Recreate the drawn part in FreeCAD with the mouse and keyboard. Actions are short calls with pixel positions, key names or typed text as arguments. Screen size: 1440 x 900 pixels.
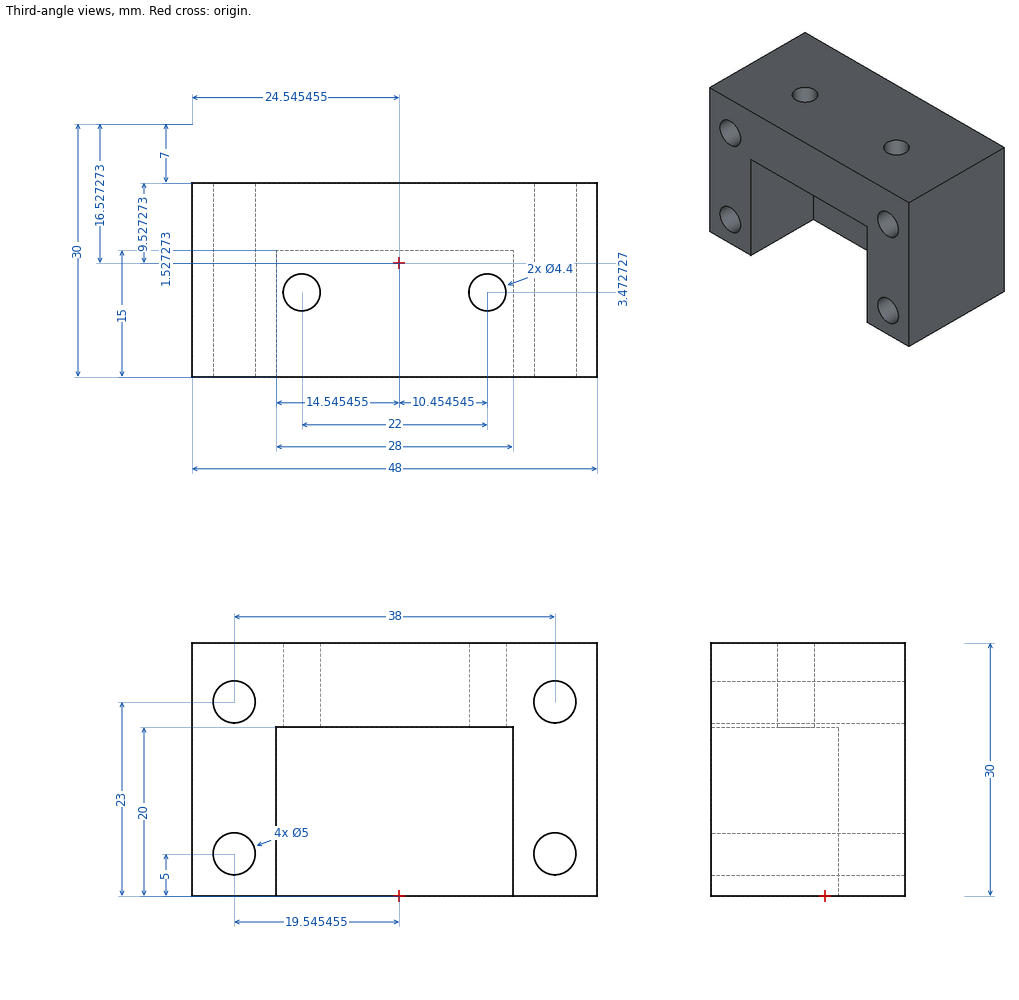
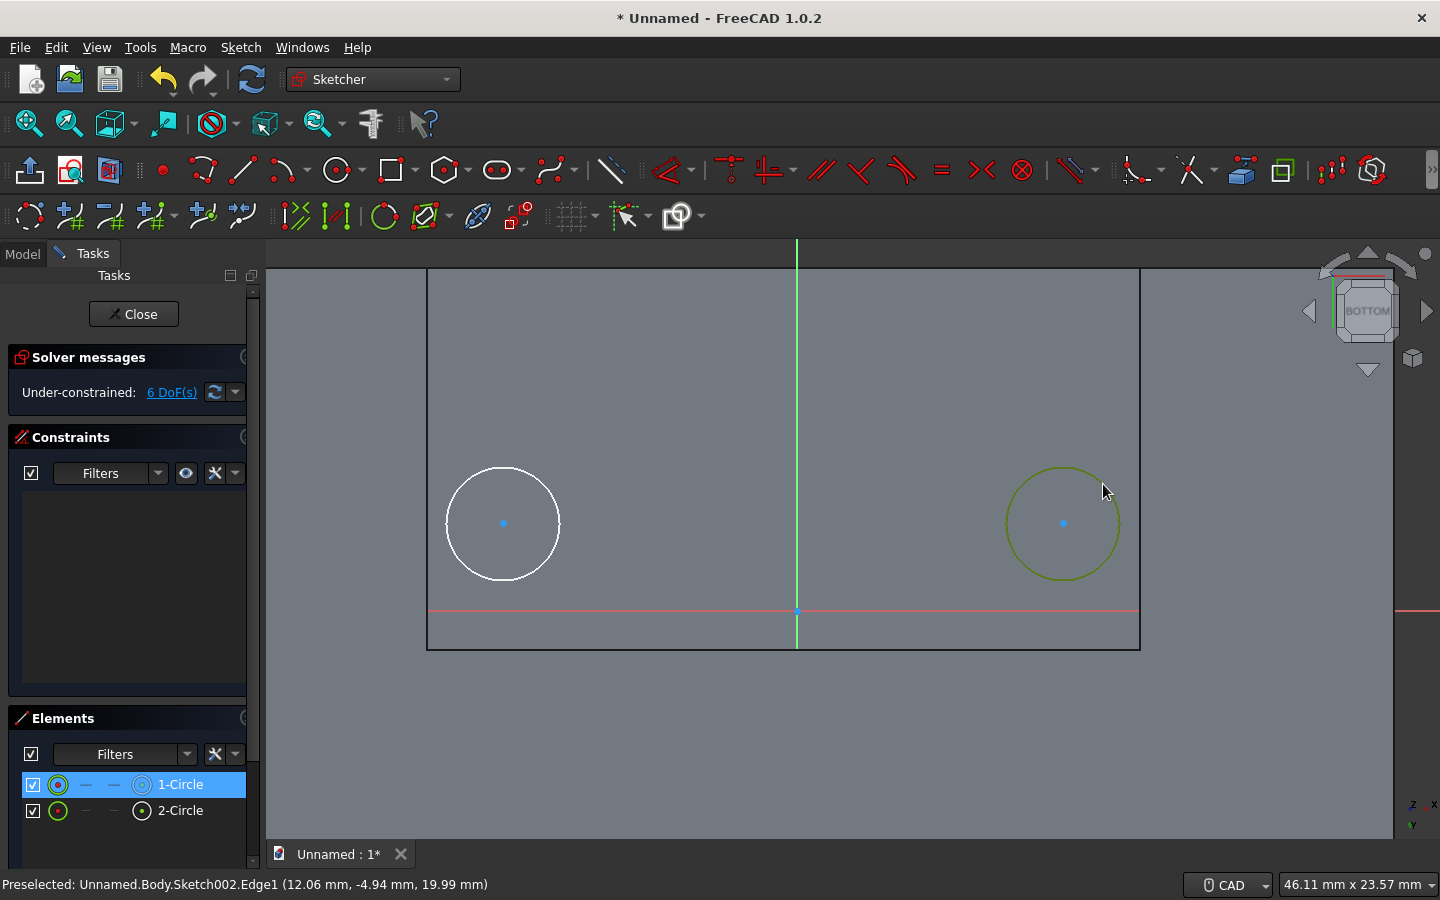
click(543, 484)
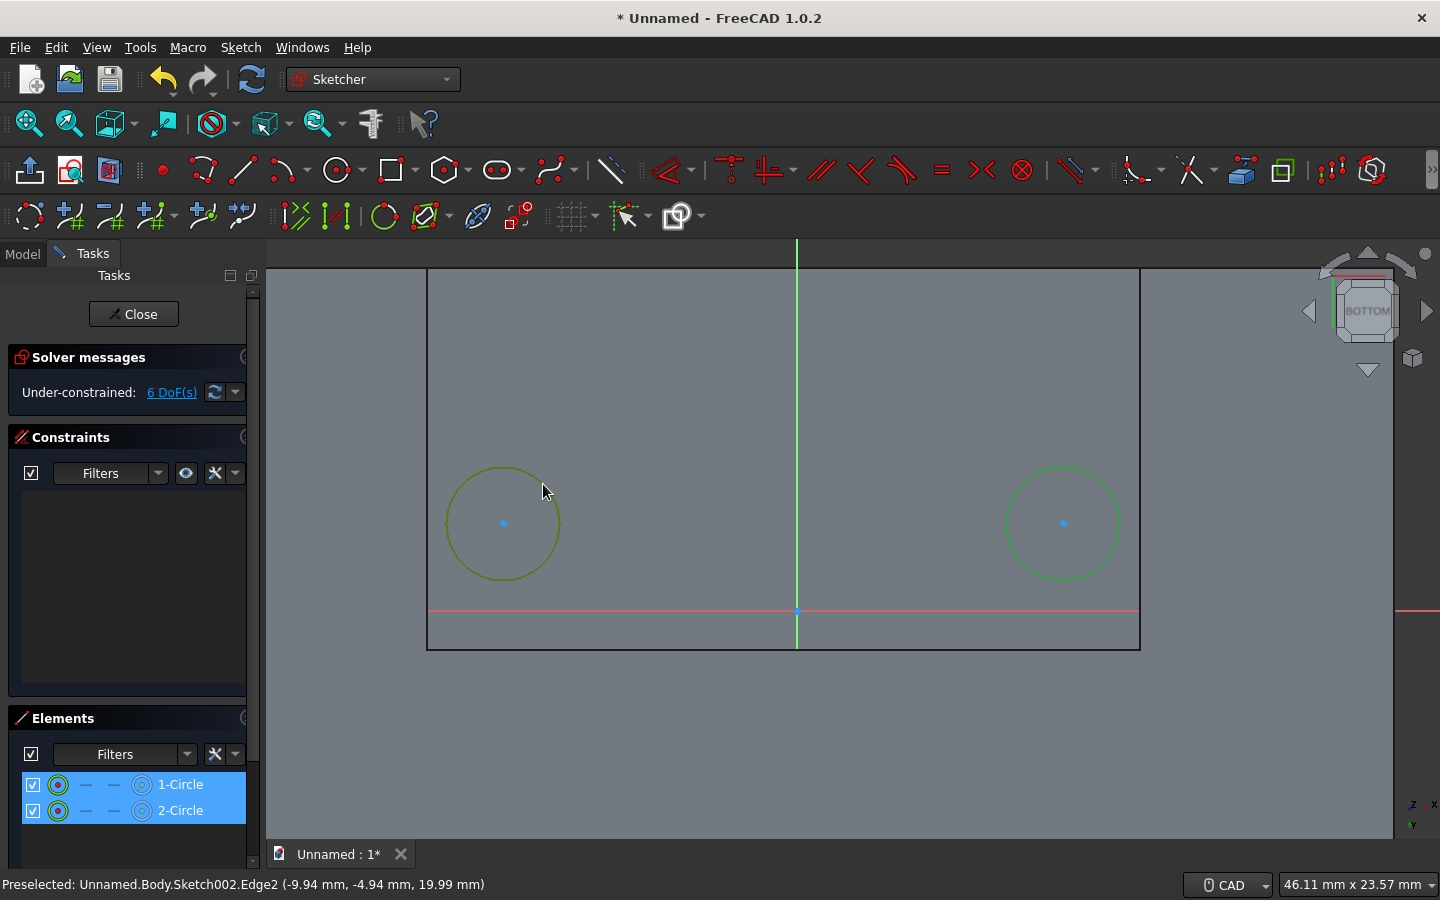
click(942, 170)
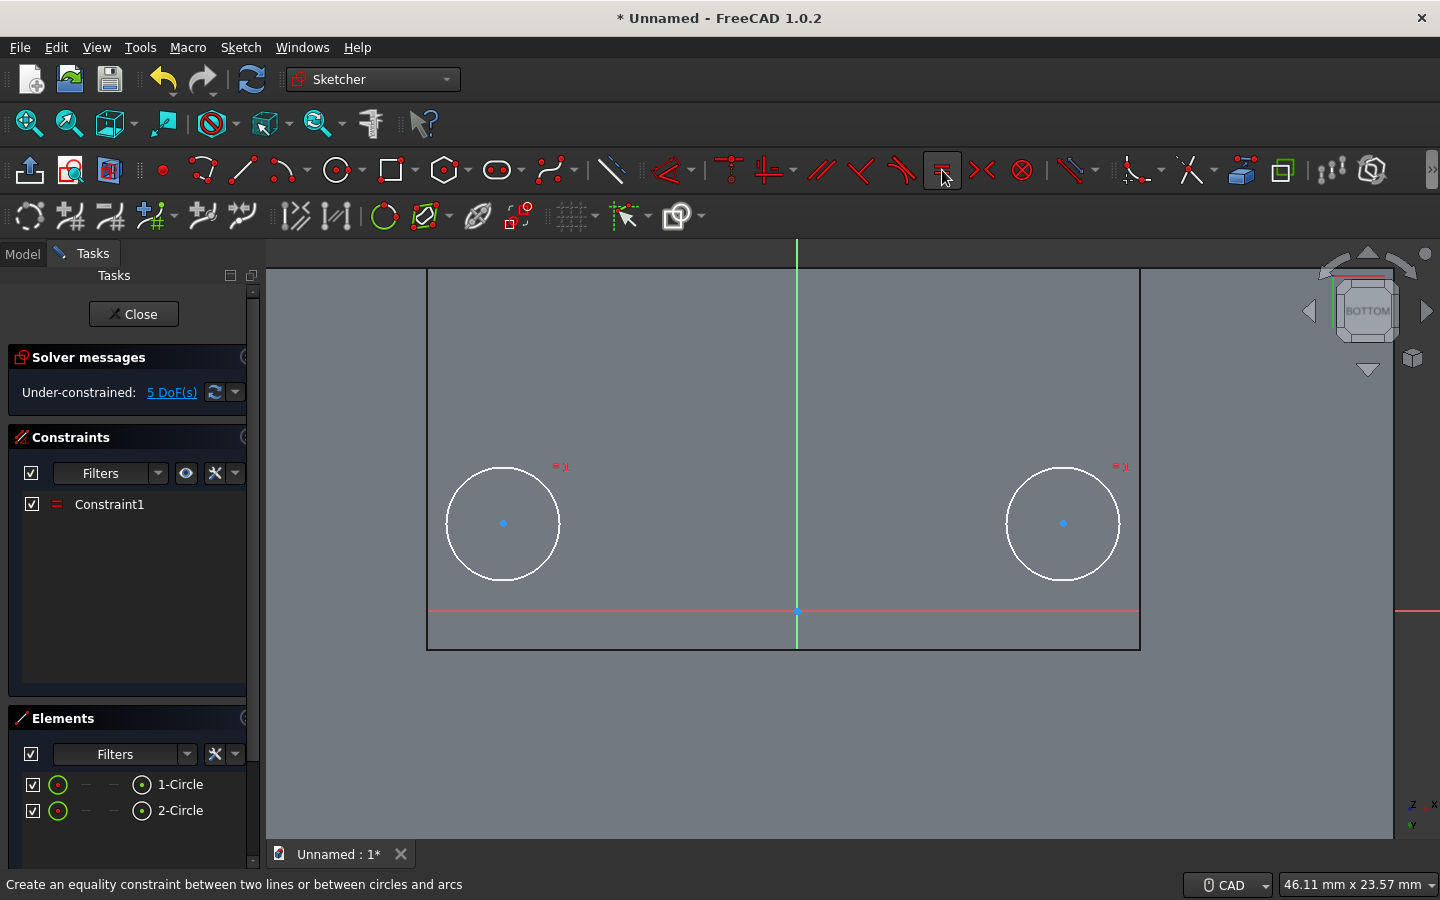
click(666, 170)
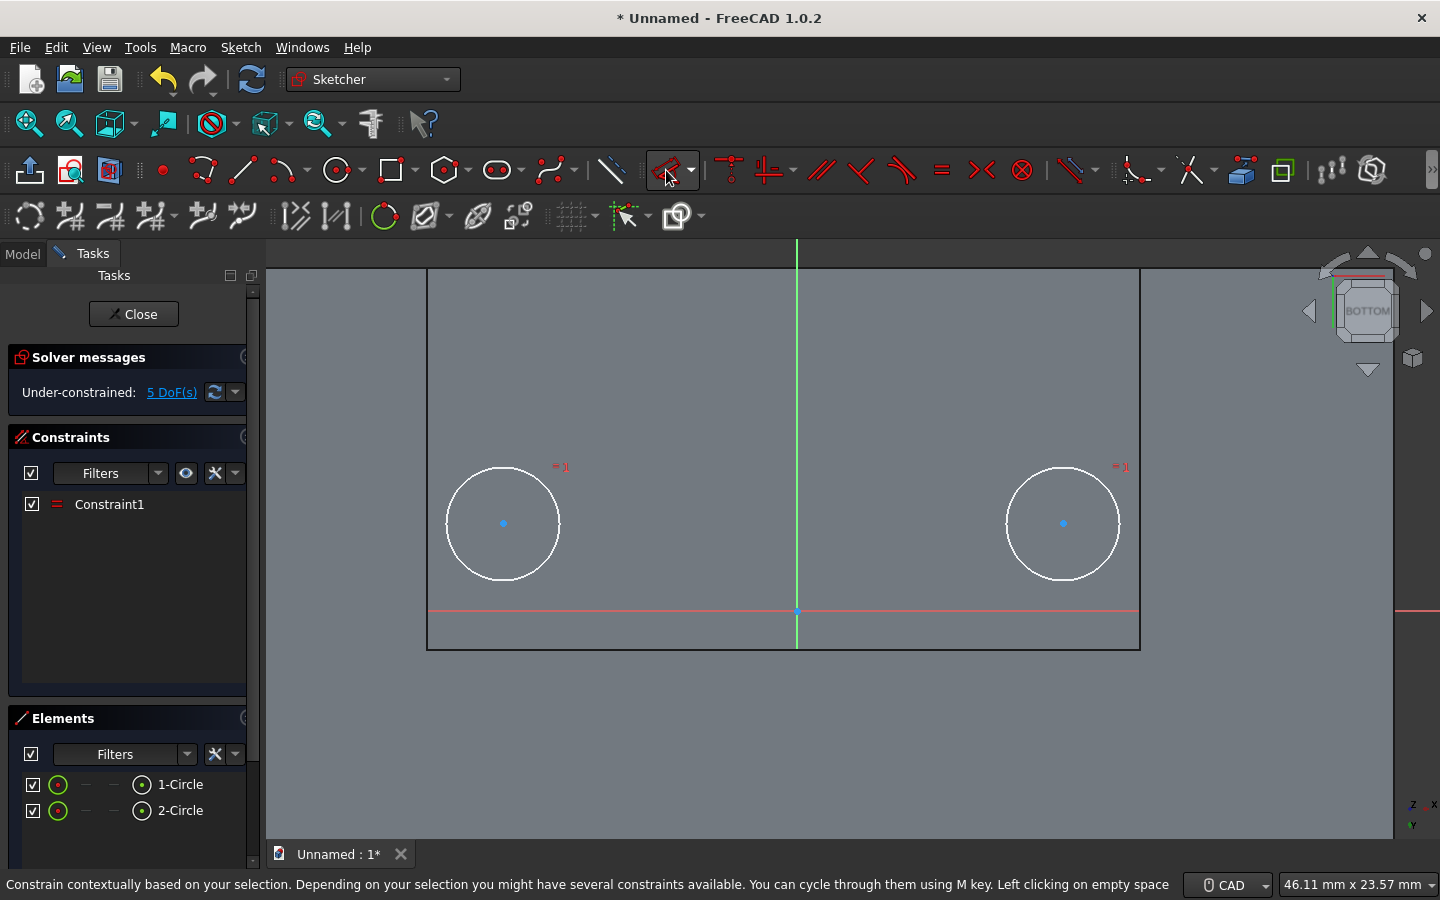
click(1103, 484)
click(1126, 461)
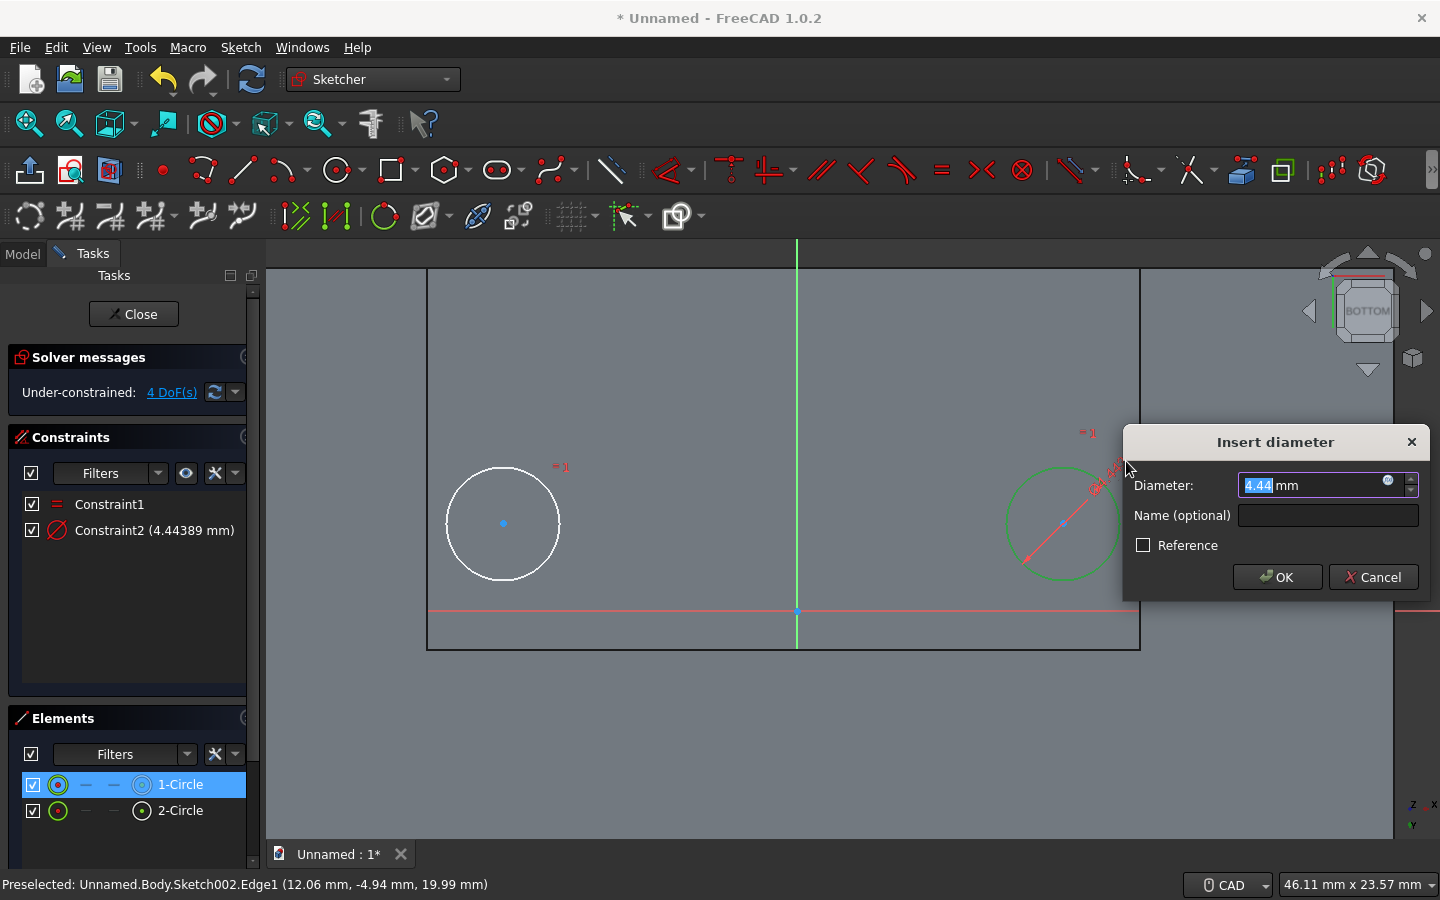
text(4.4)
key(Return)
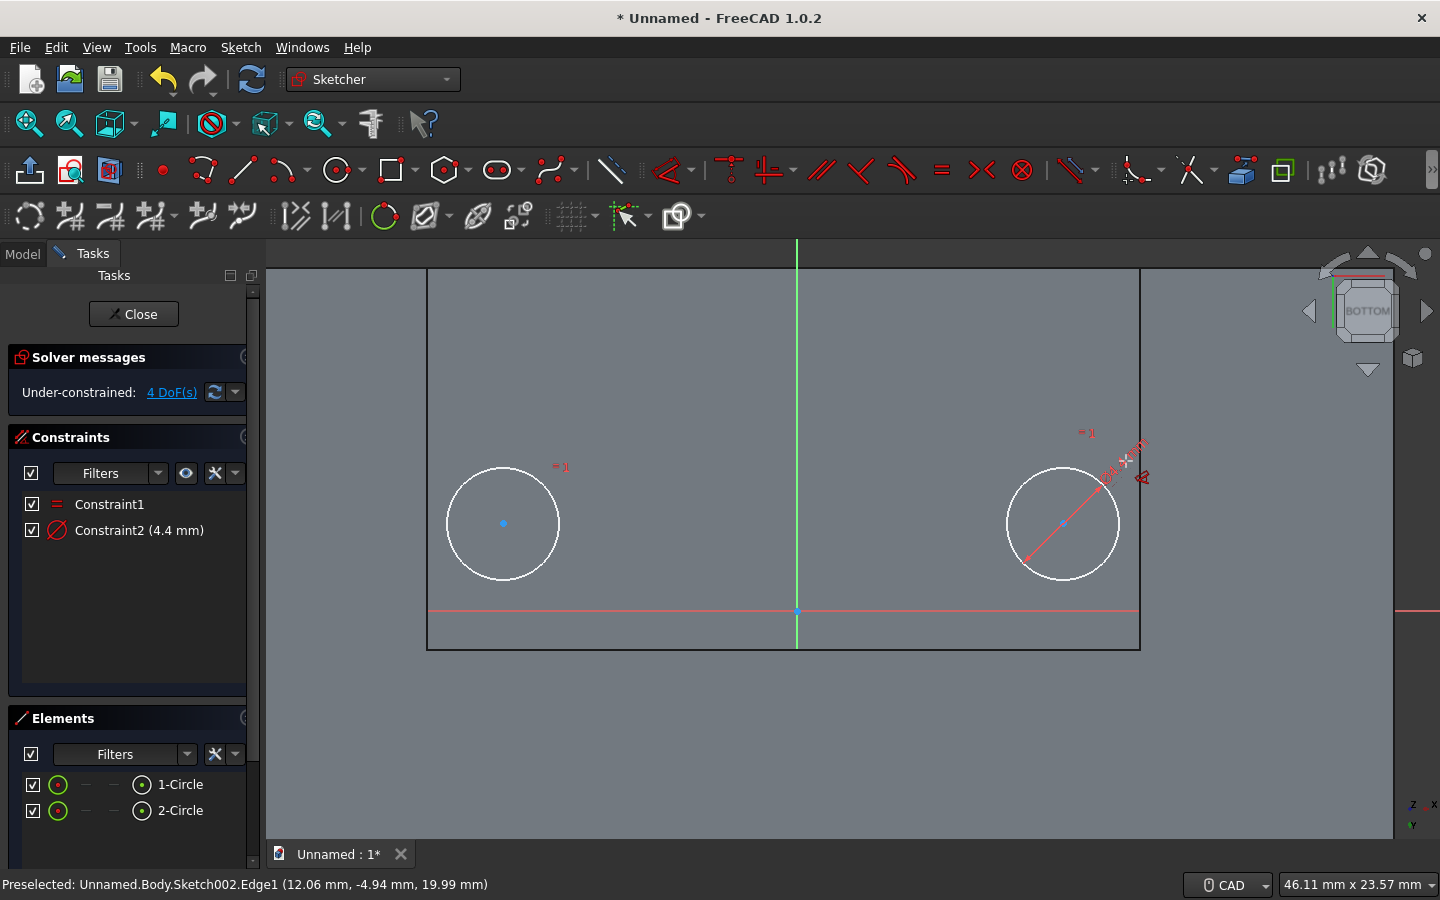
click(1063, 524)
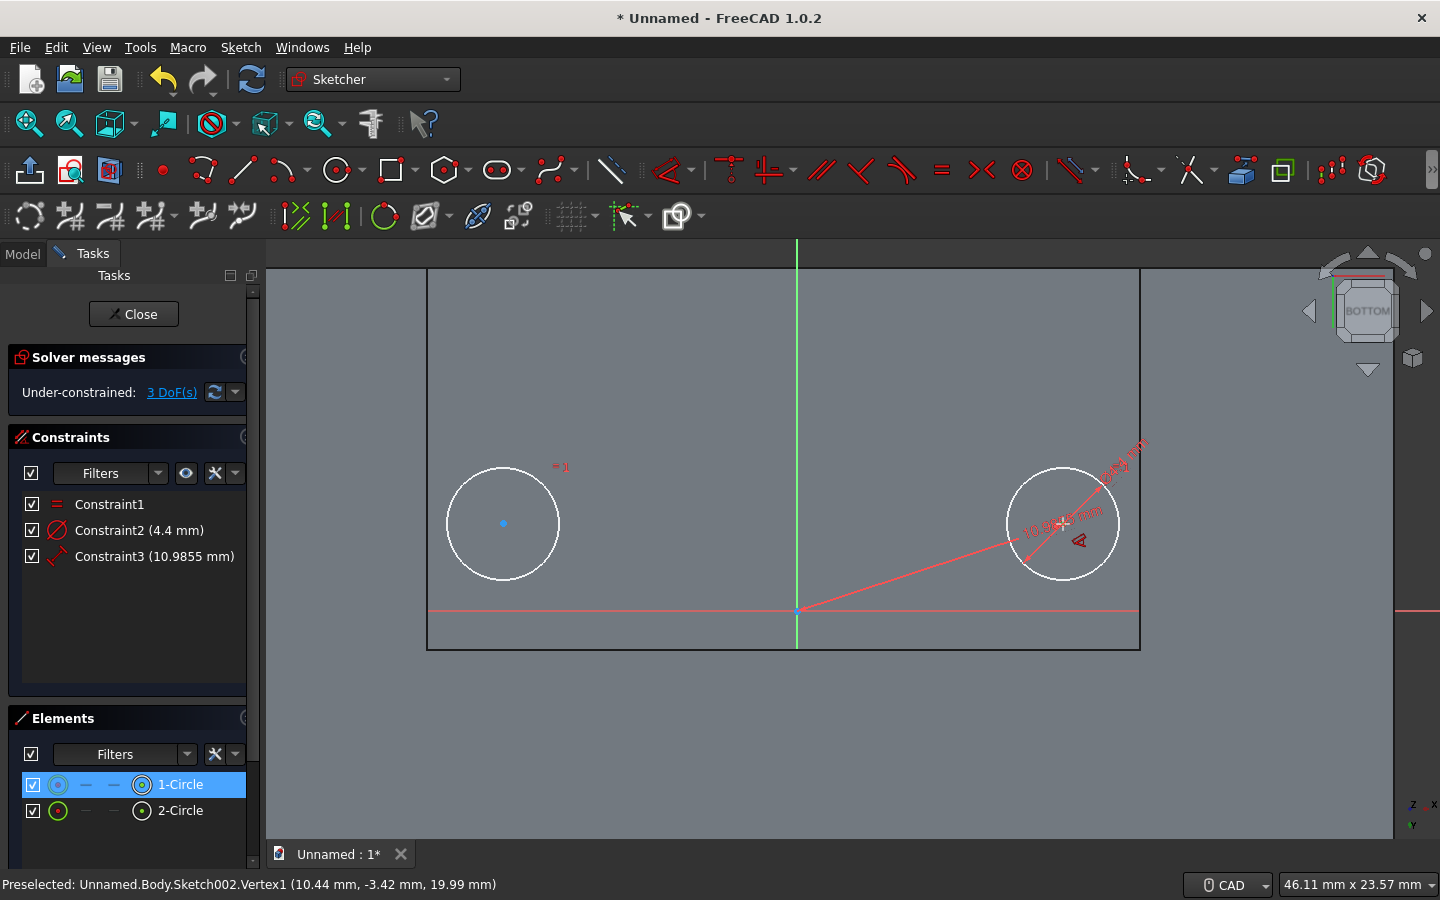
click(503, 524)
click(783, 490)